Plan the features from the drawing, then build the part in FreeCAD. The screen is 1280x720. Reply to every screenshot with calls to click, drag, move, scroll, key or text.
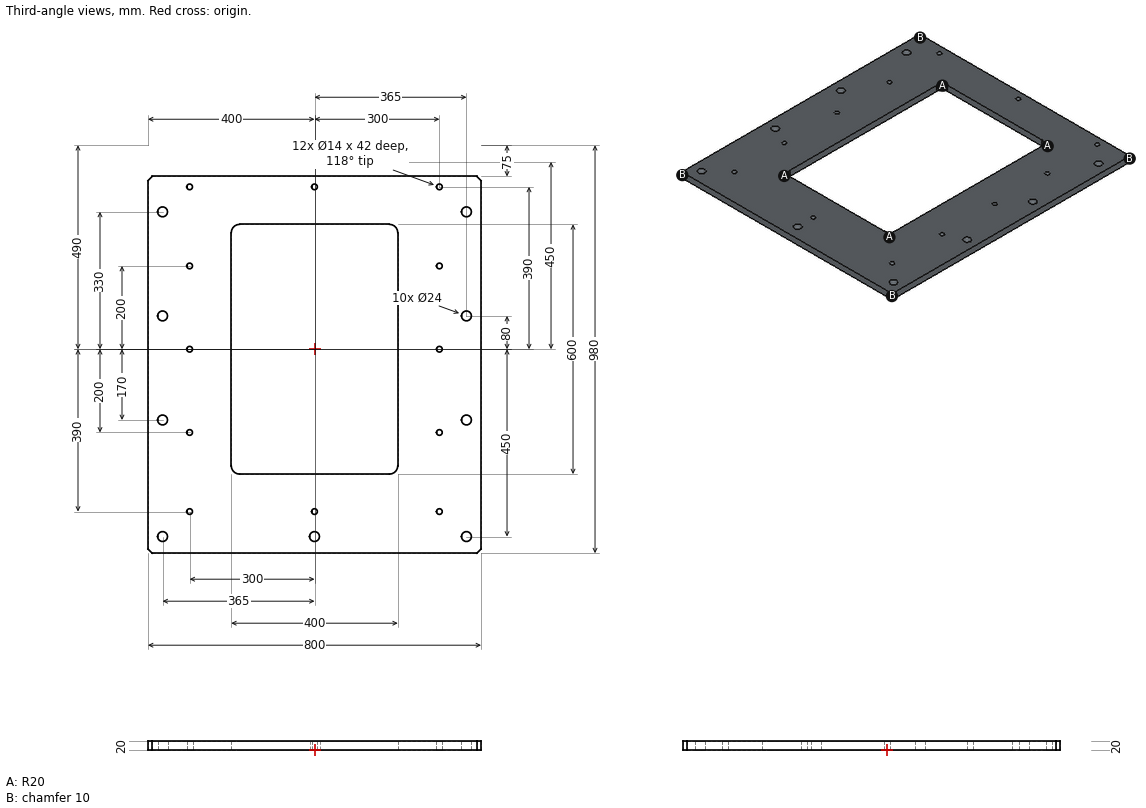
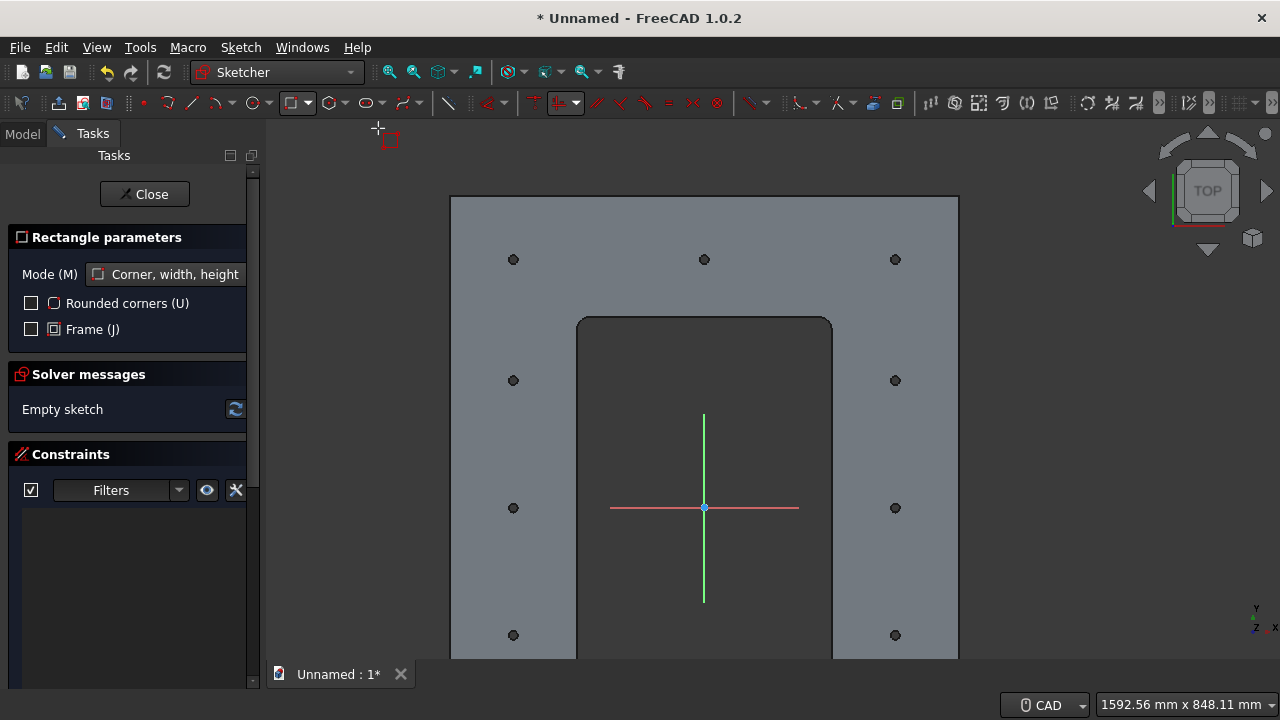
click(450, 196)
move(959, 244)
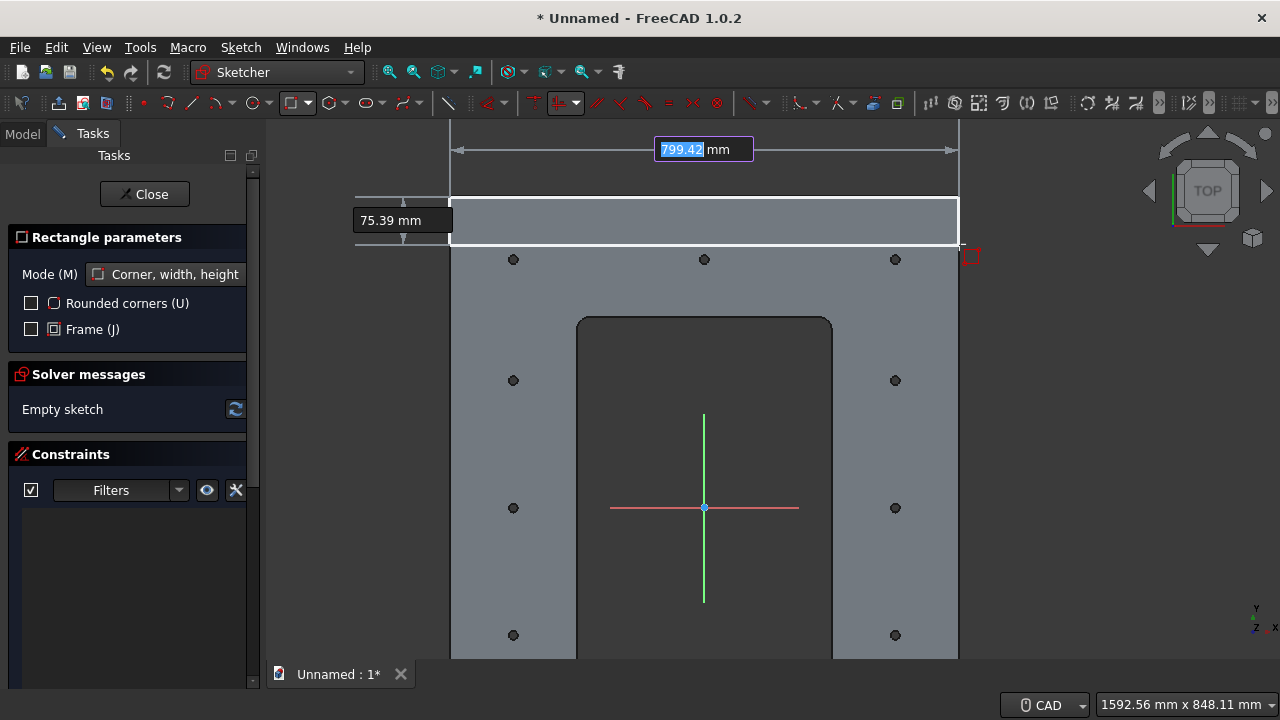
text(800)
key(Tab)
text(75)
key(Return)
key(Escape)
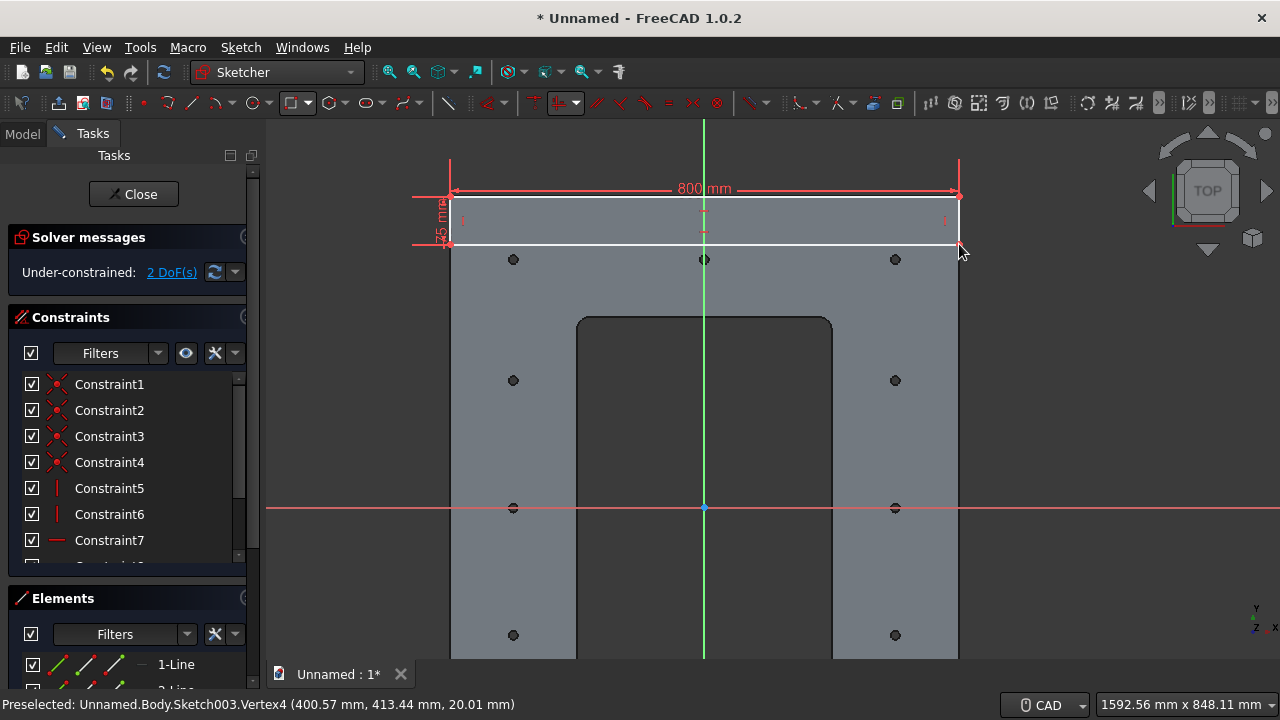
click(488, 104)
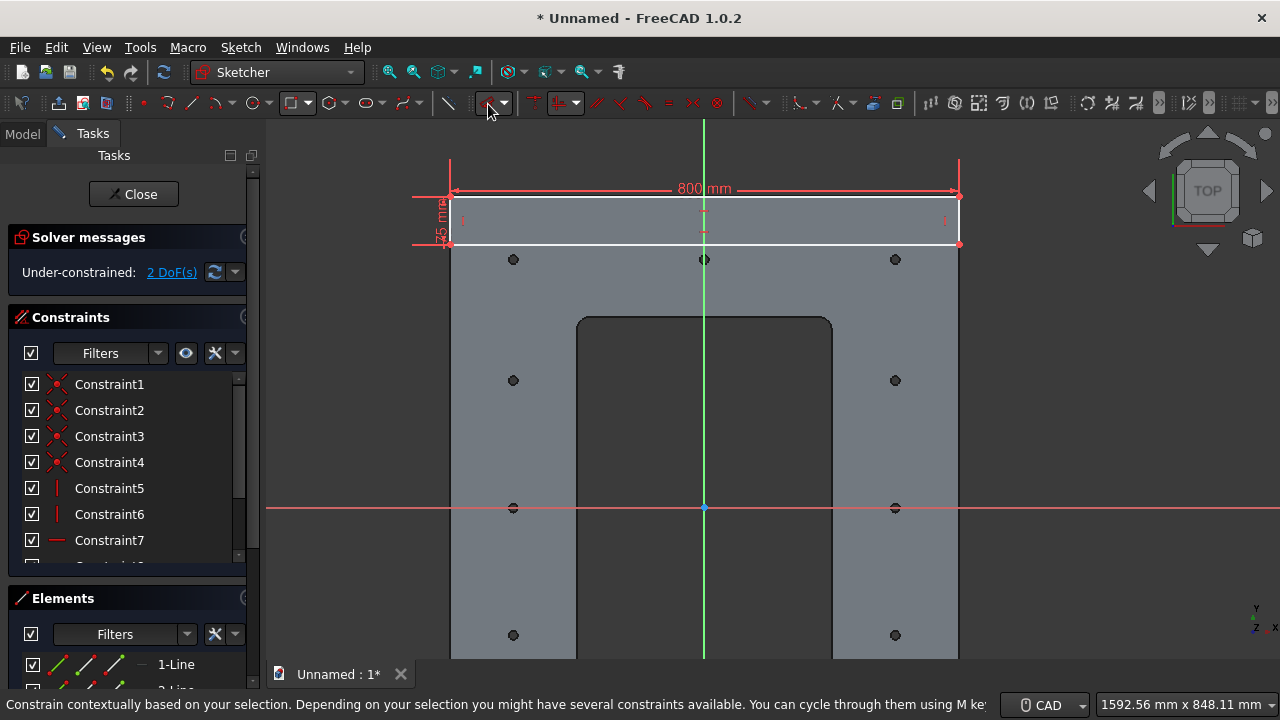
click(450, 197)
click(577, 542)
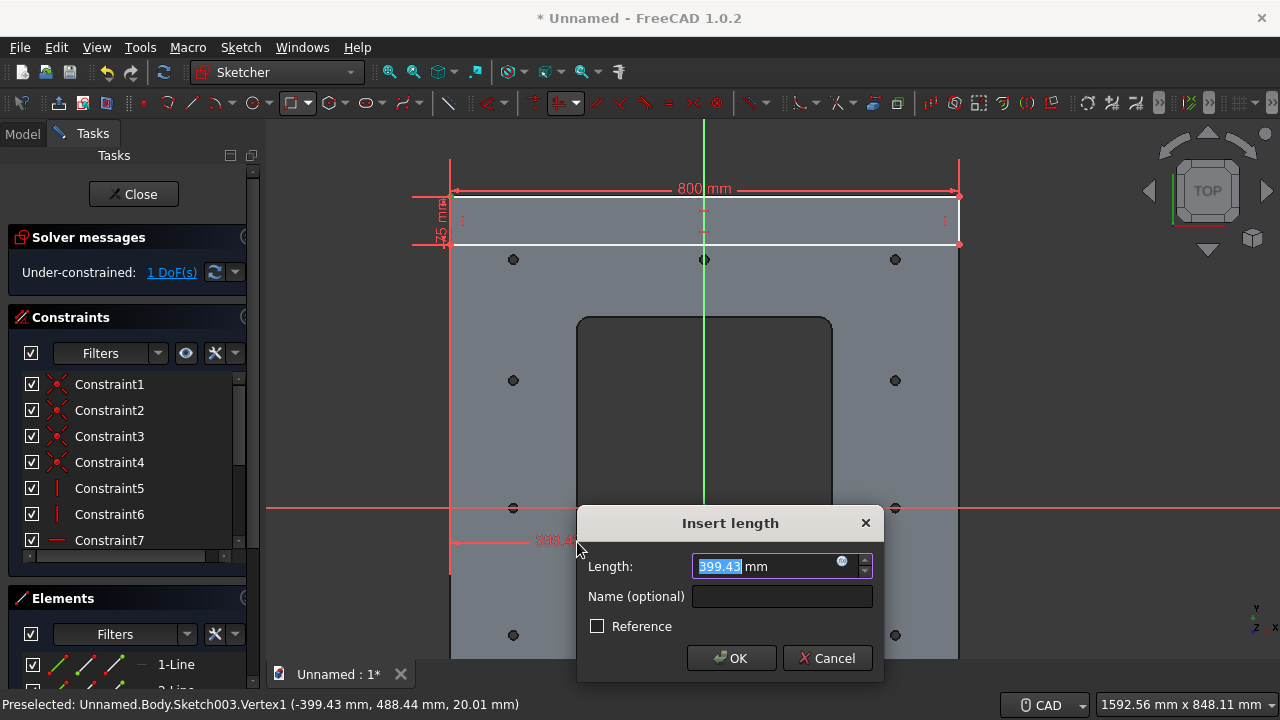
text(400)
key(Return)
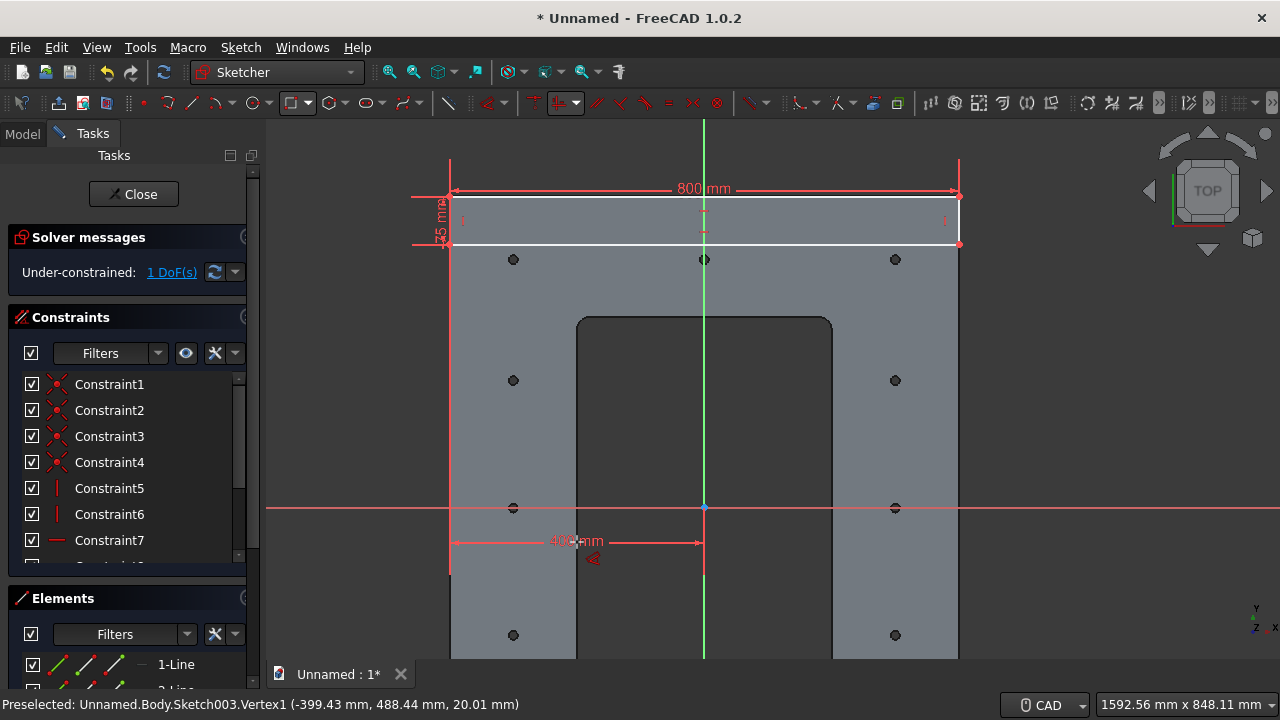
click(450, 197)
click(416, 352)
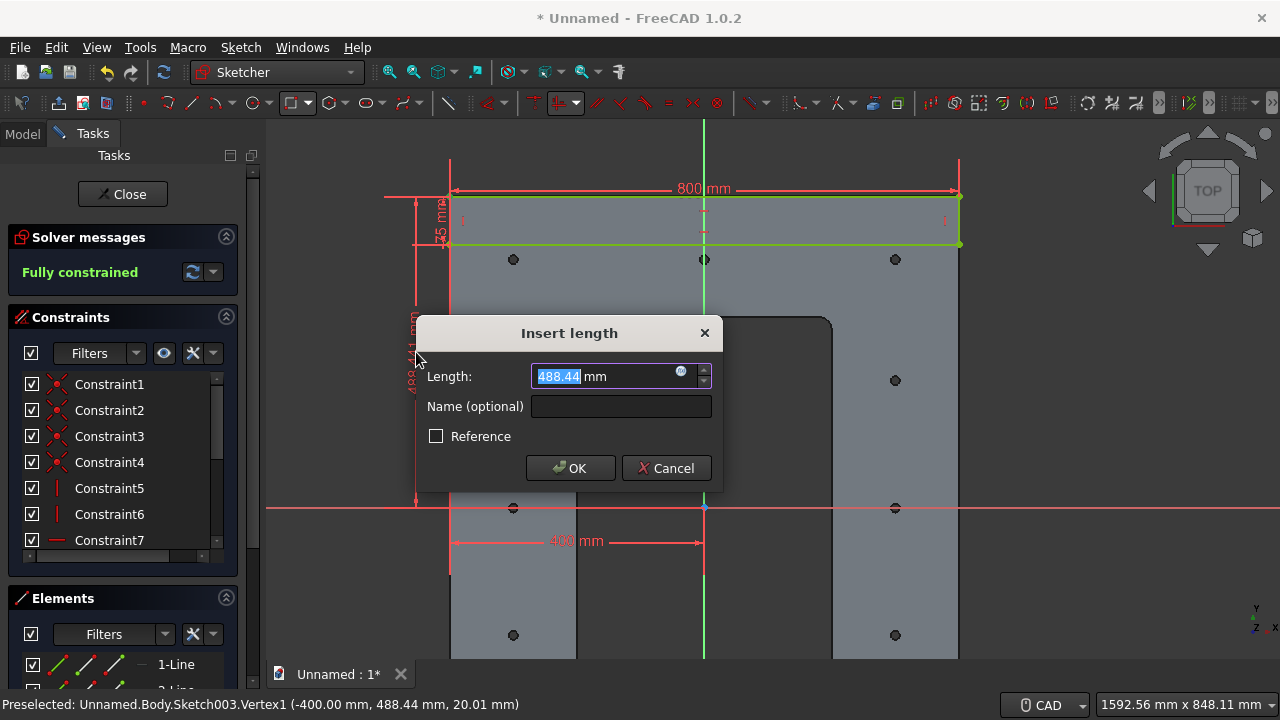
text(490)
key(Return)
key(Escape)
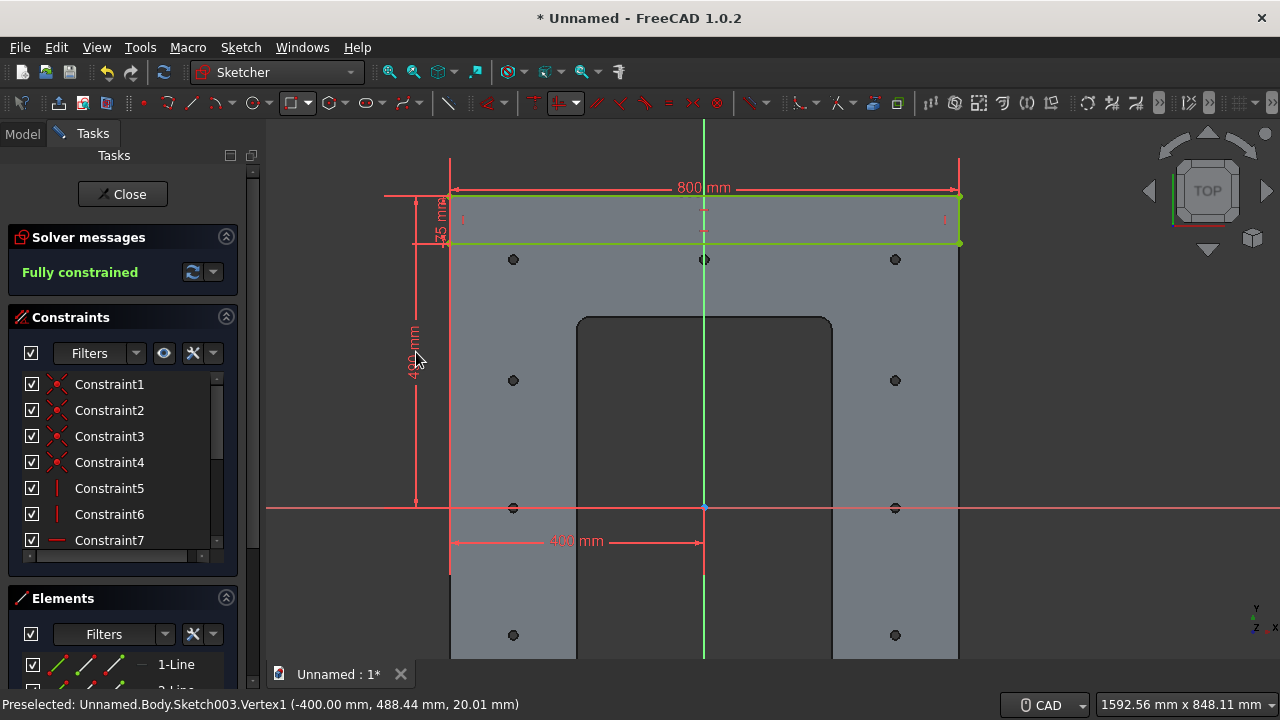
click(123, 194)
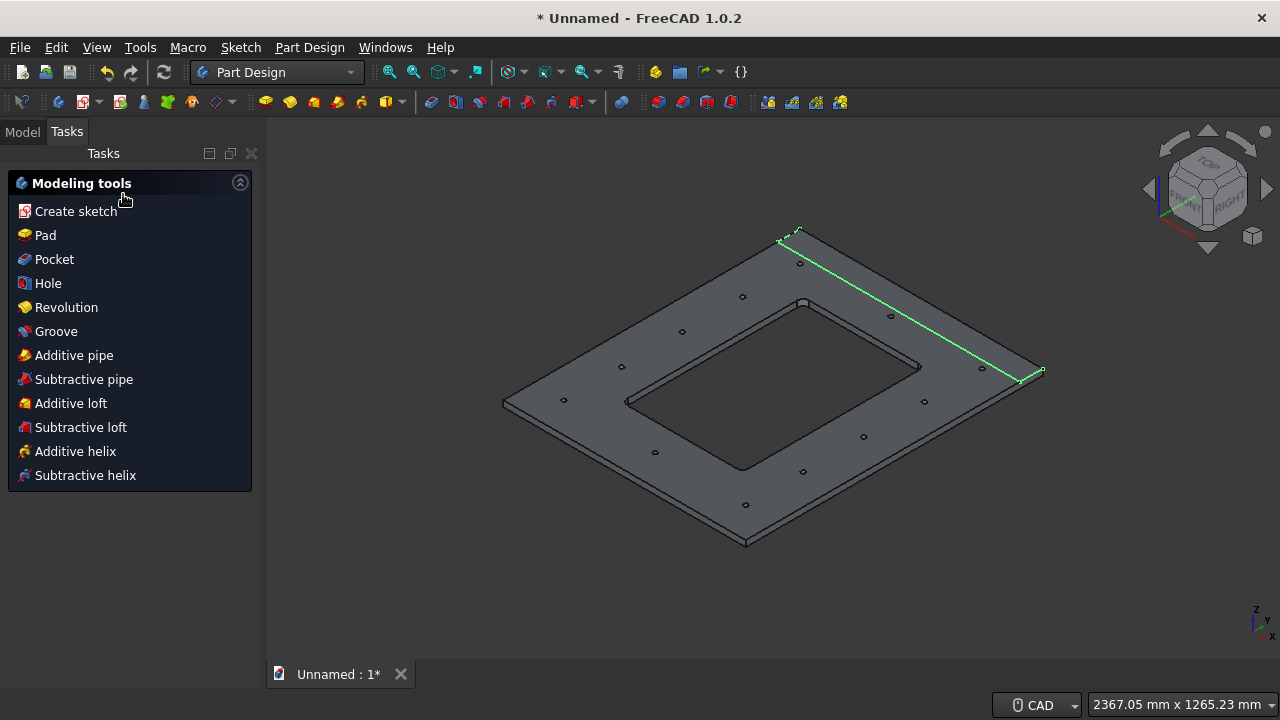
click(432, 102)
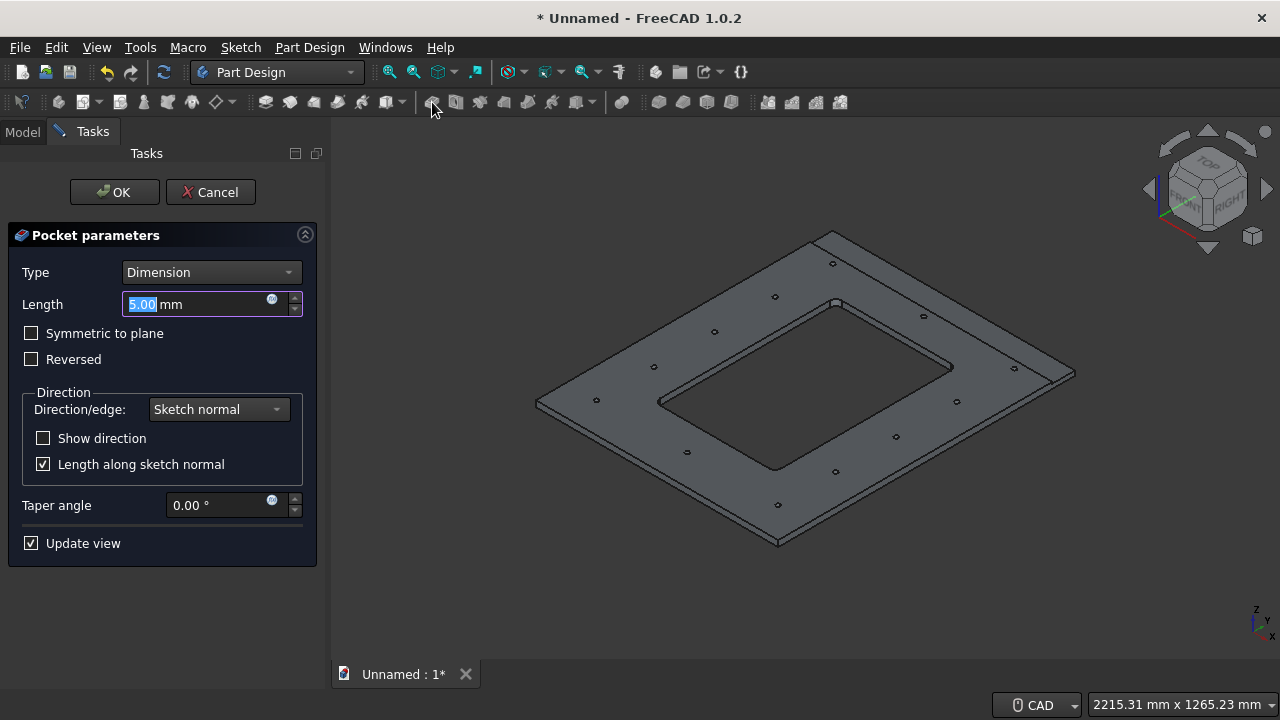
click(212, 272)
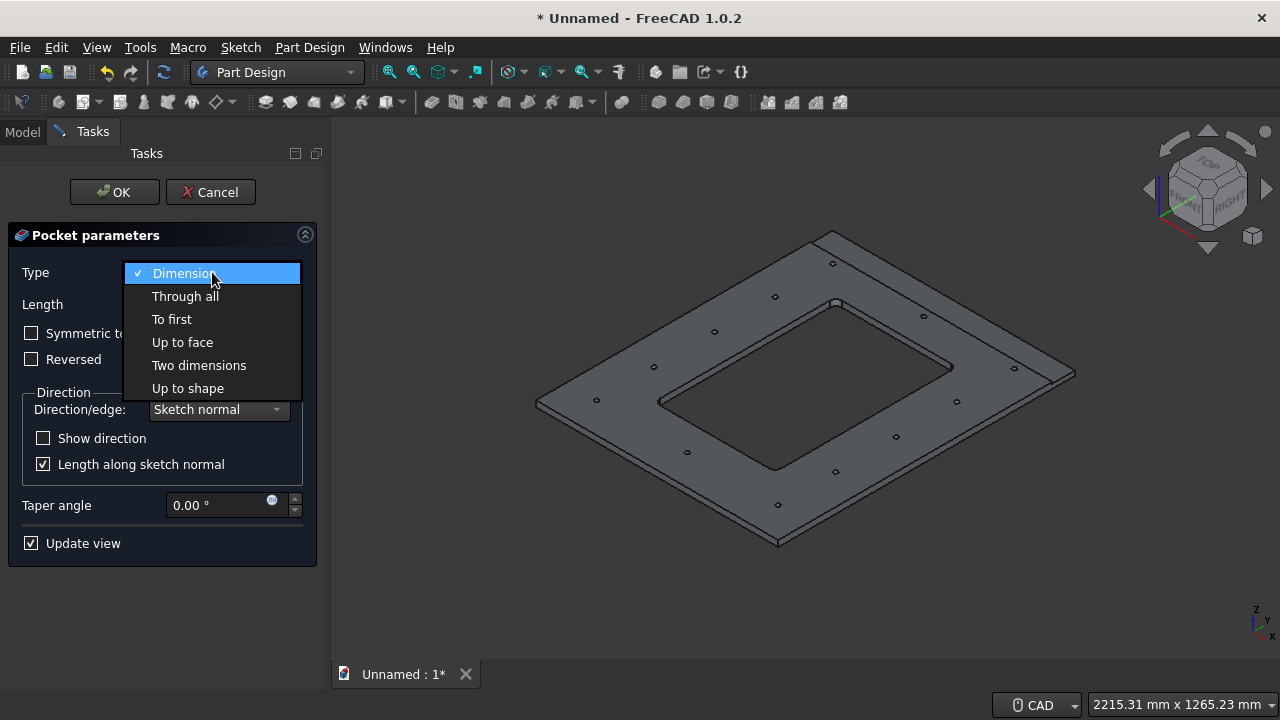
click(212, 296)